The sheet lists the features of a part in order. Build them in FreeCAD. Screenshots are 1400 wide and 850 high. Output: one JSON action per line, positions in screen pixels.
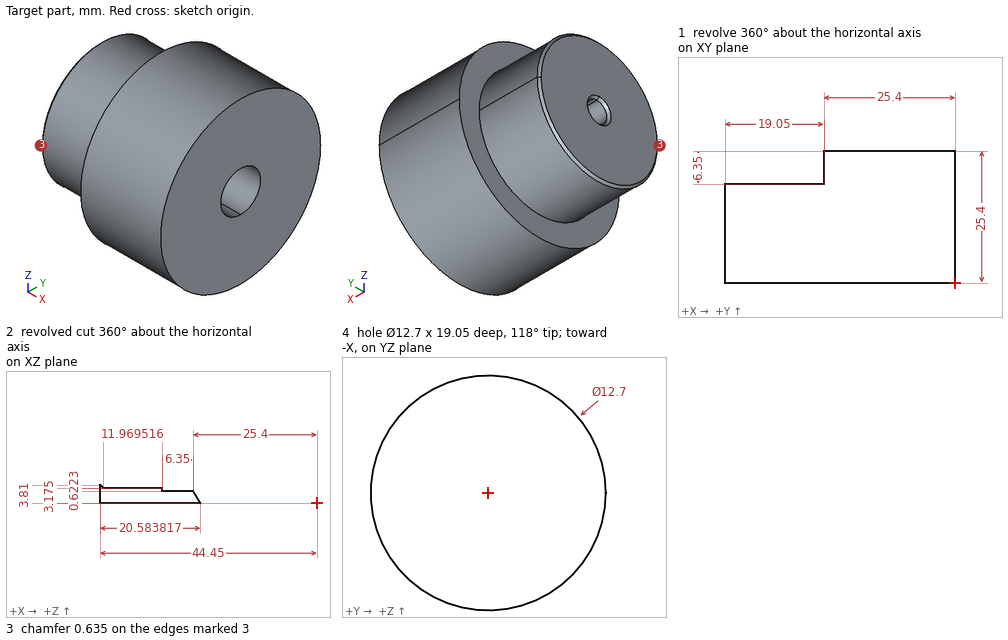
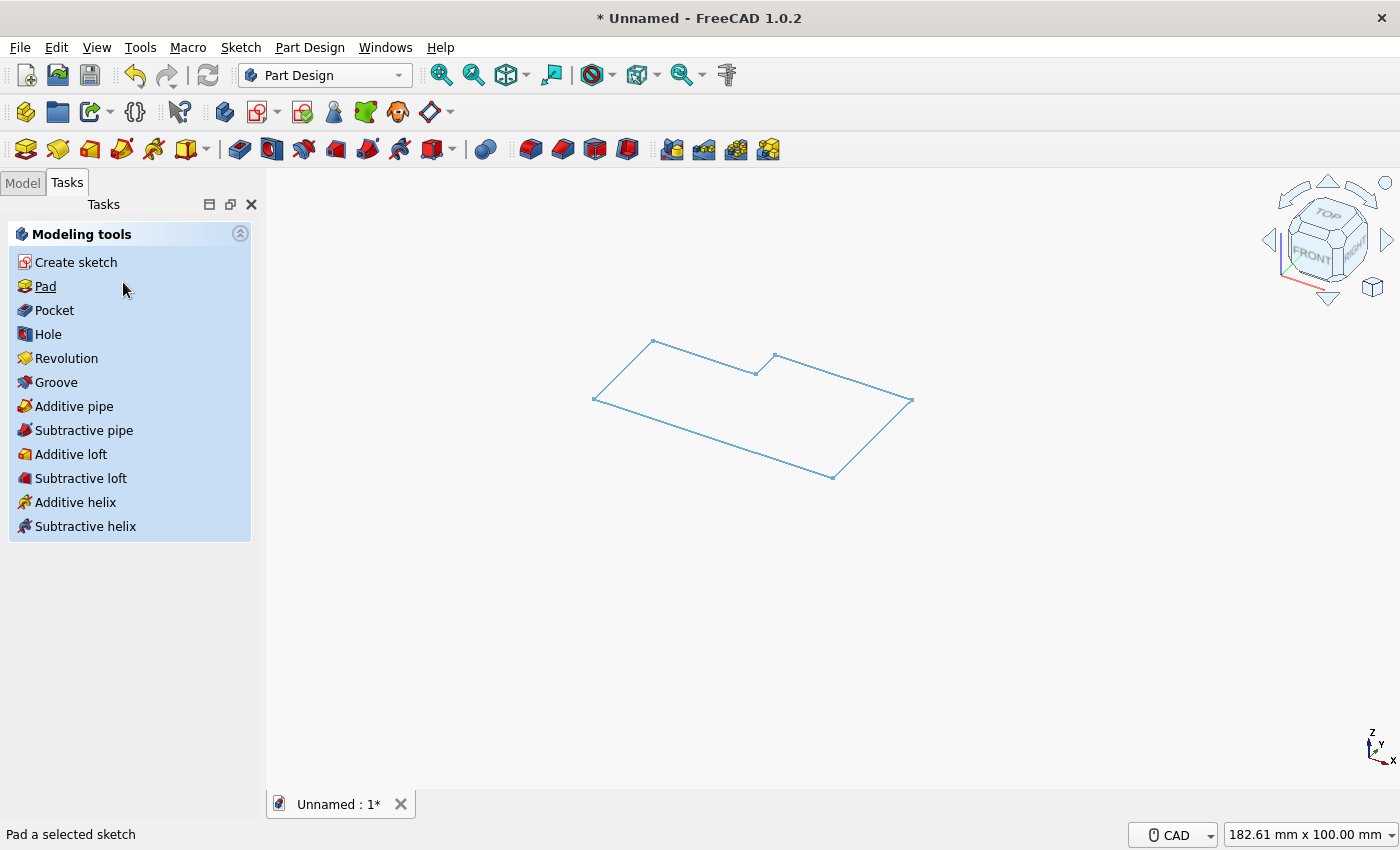
{"action": "left_click", "coordinate": [58, 150]}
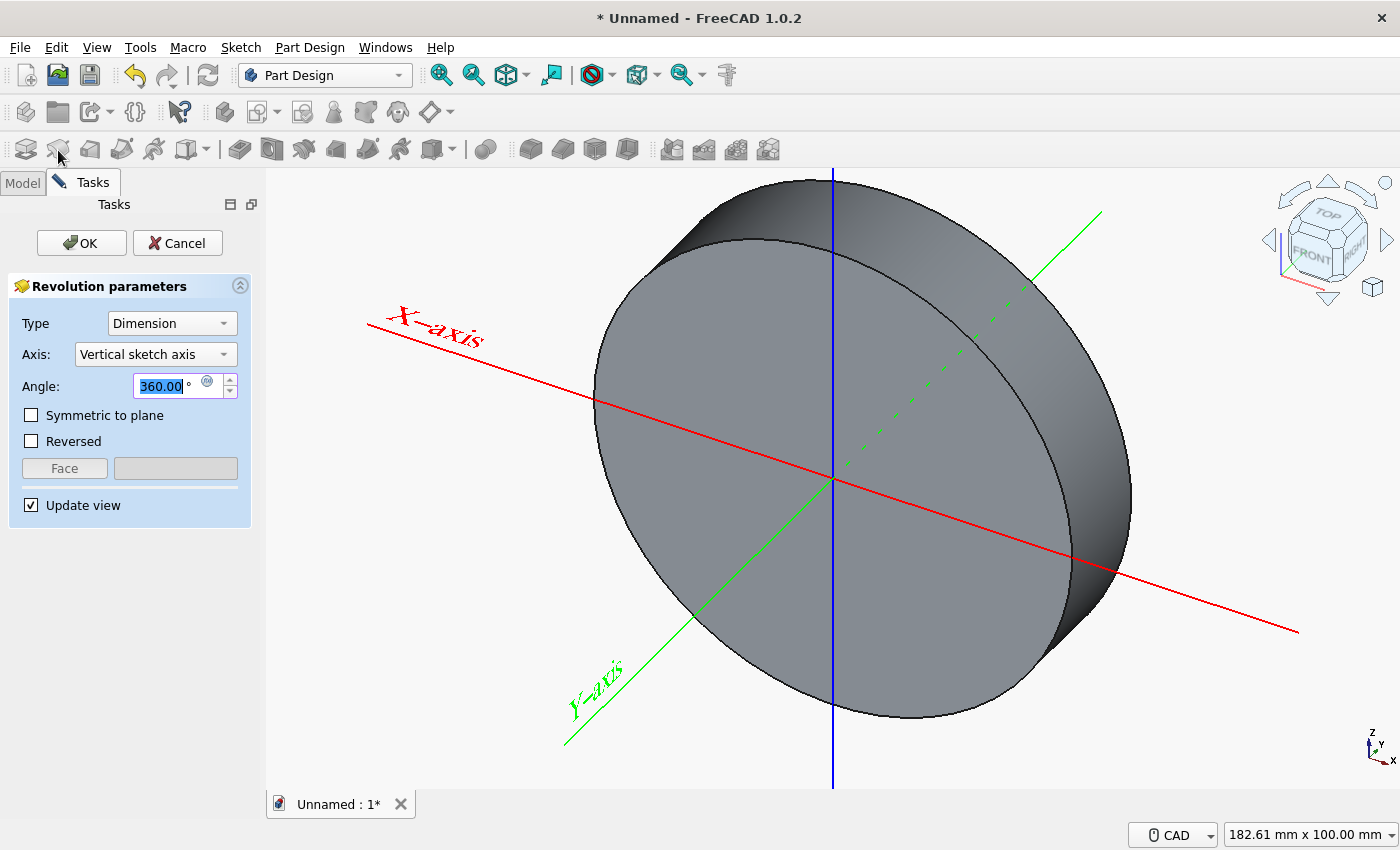
{"action": "left_click", "coordinate": [156, 354]}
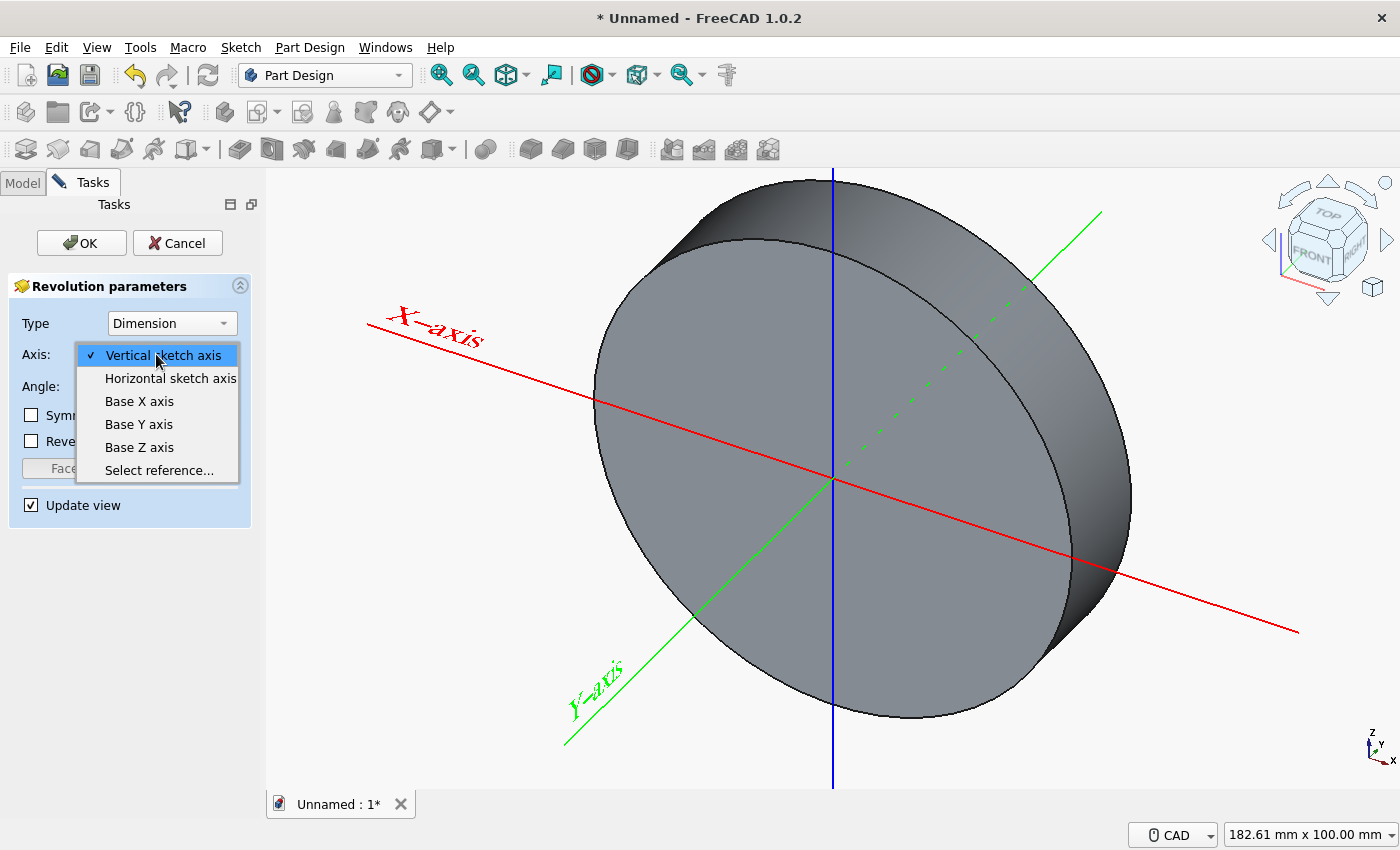
{"action": "left_click", "coordinate": [156, 378]}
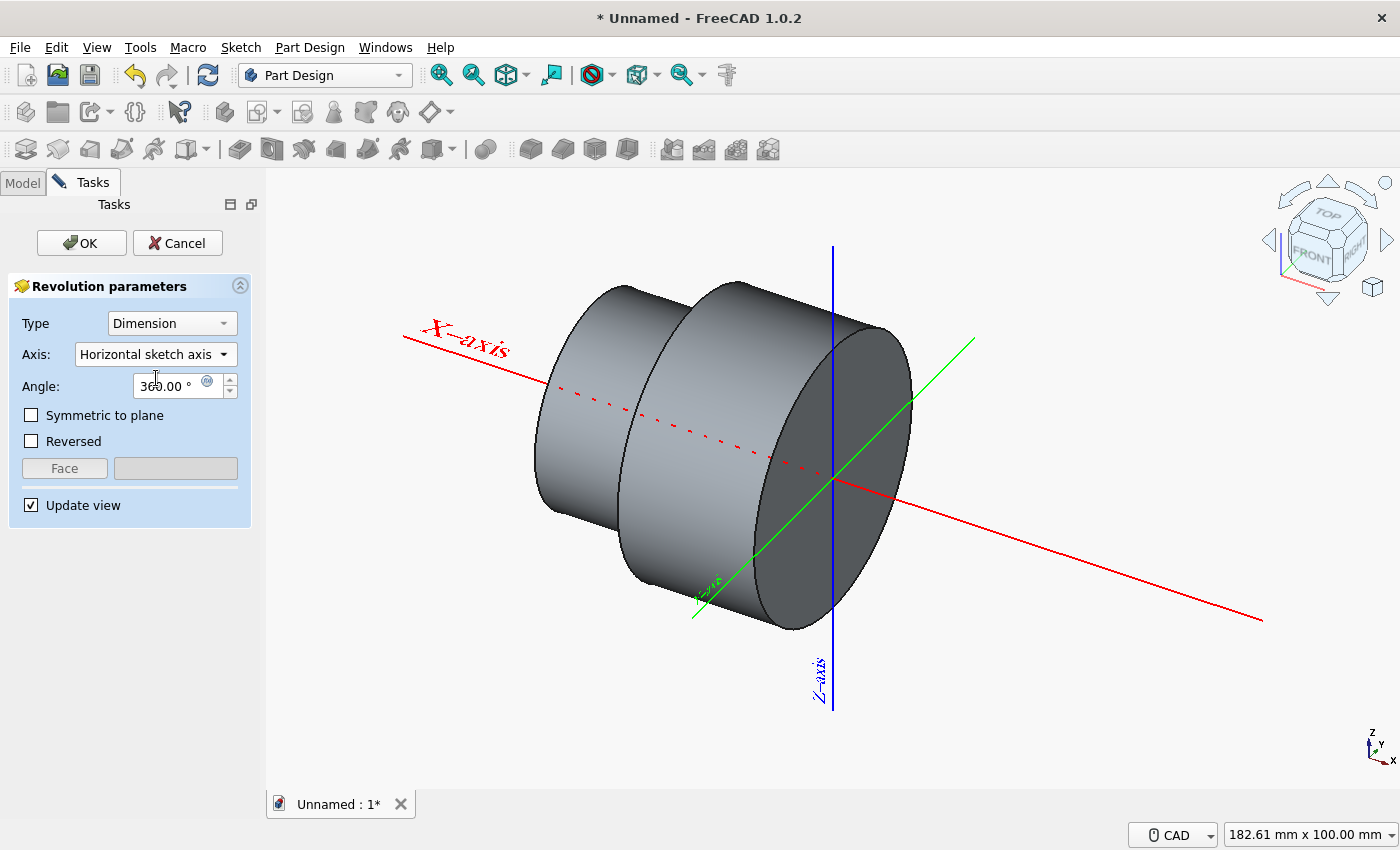
{"action": "left_click", "coordinate": [82, 243]}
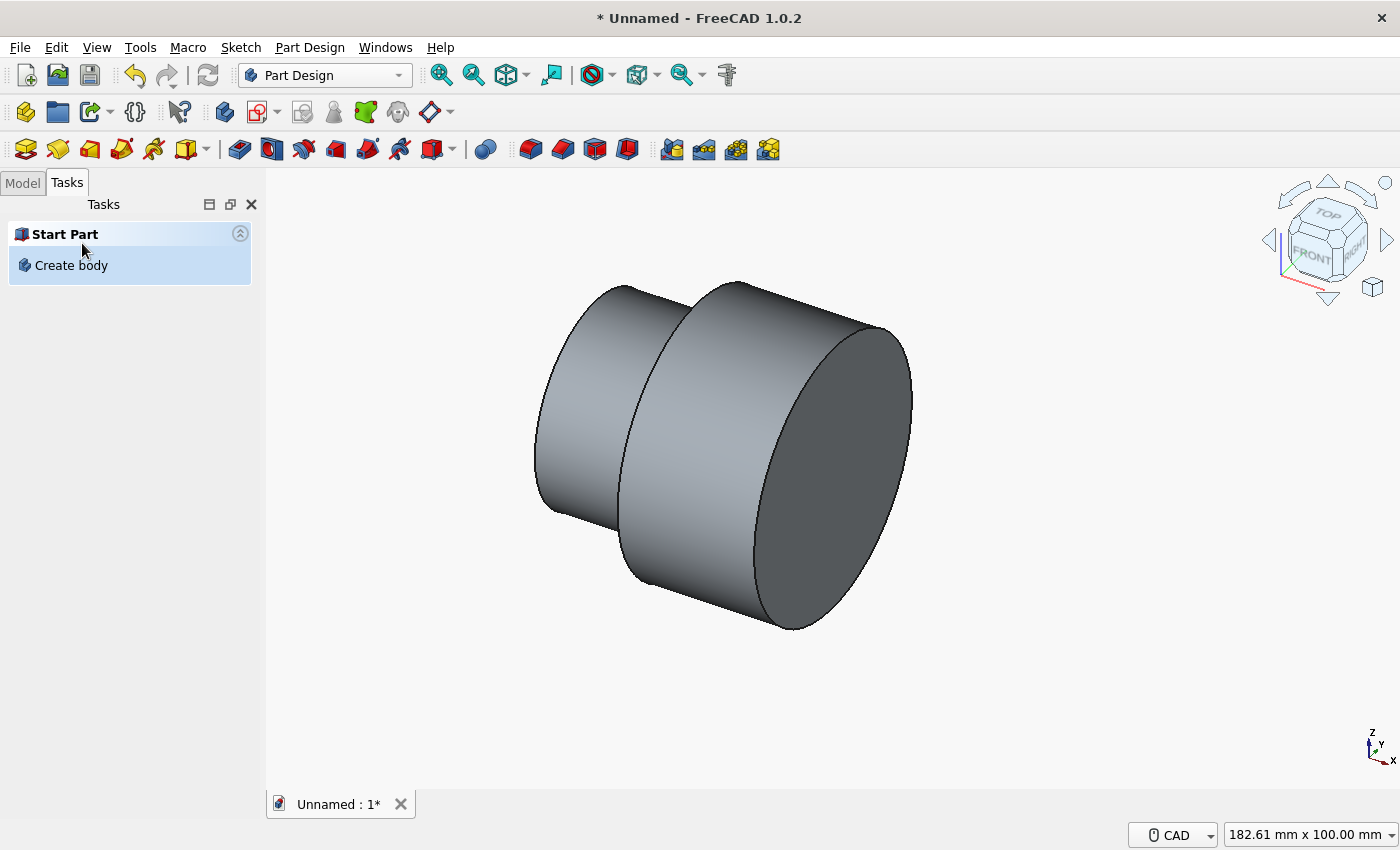
{"action": "left_click", "coordinate": [258, 112]}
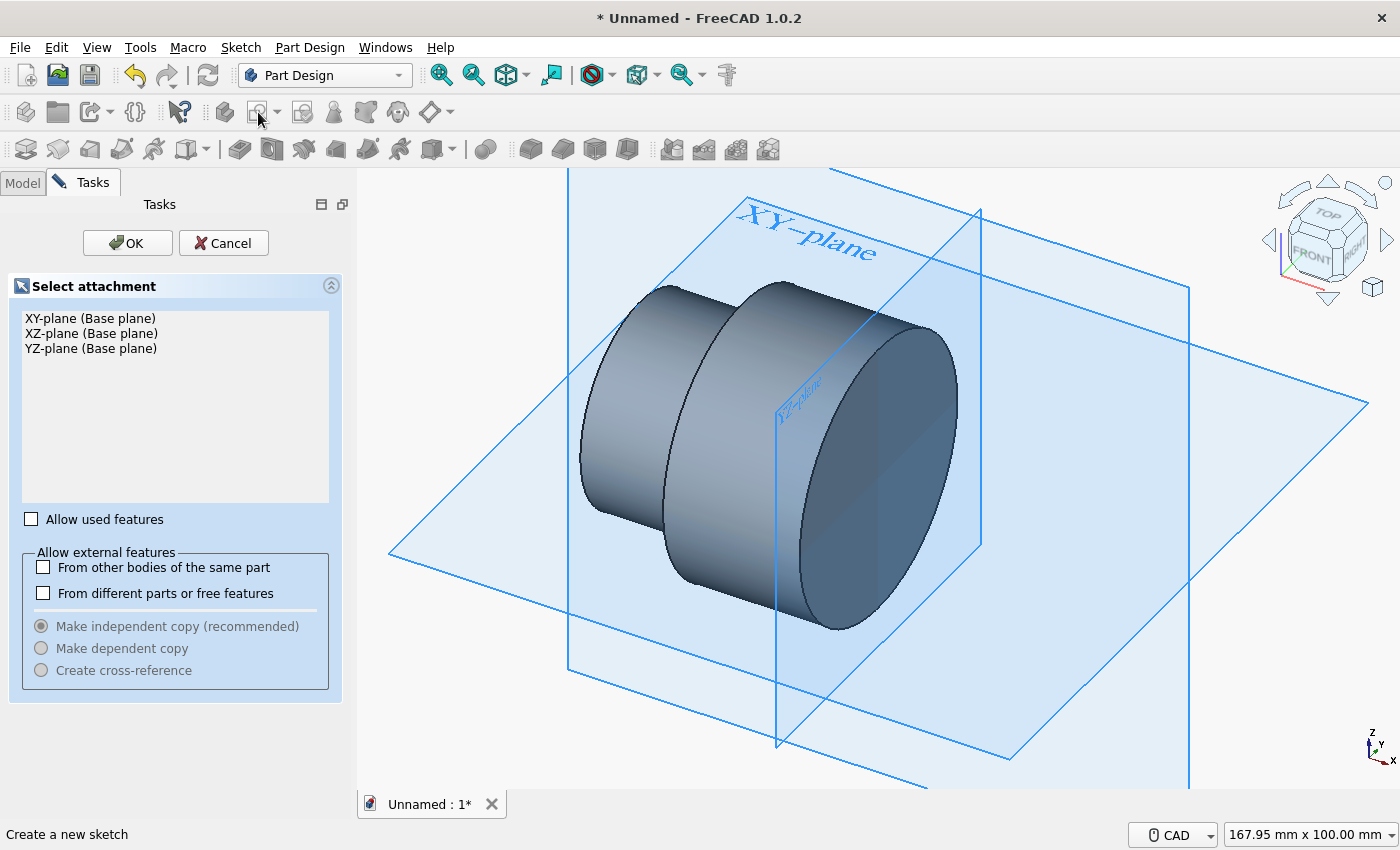
{"action": "left_click", "coordinate": [82, 334]}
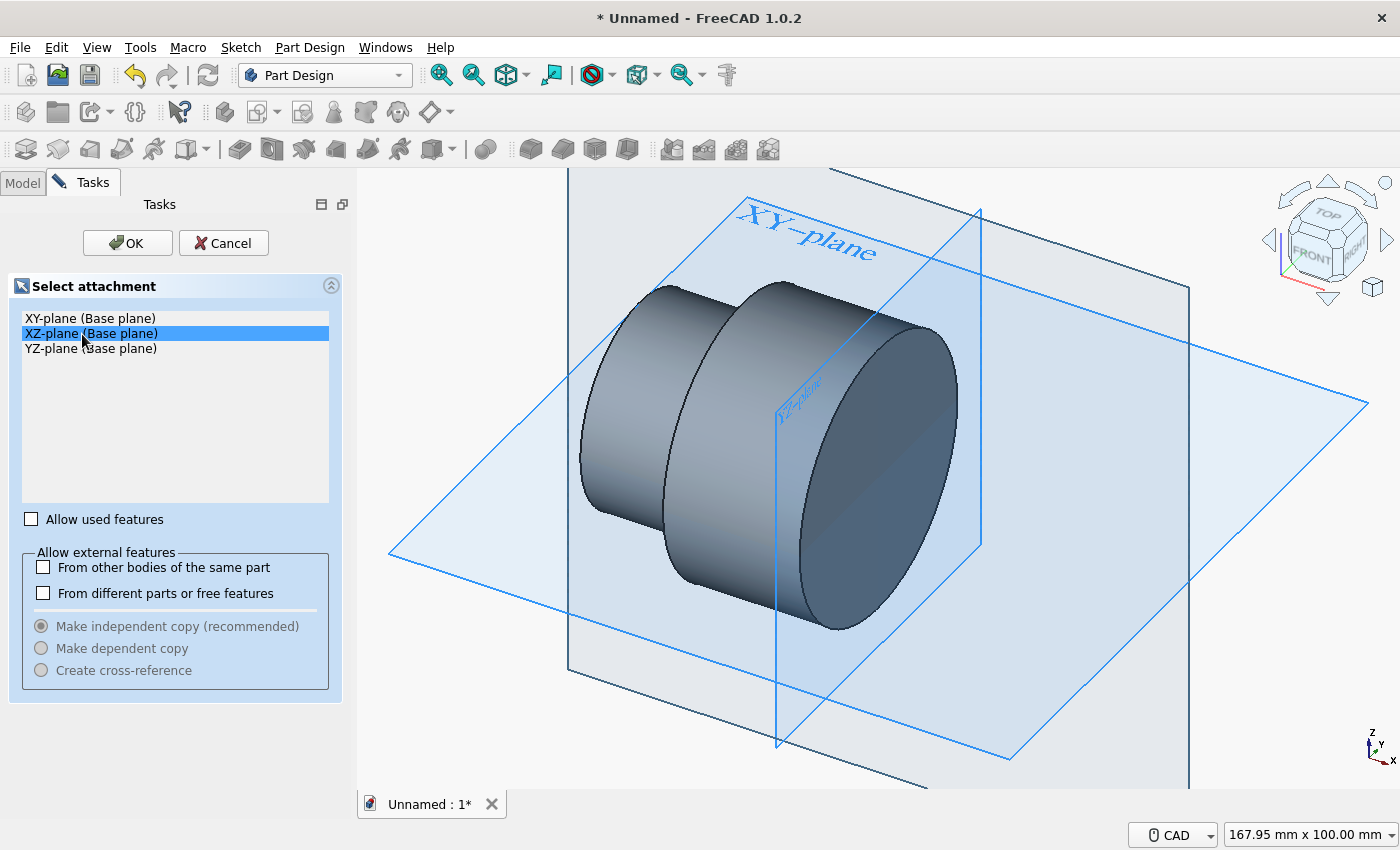
{"action": "left_click", "coordinate": [128, 243]}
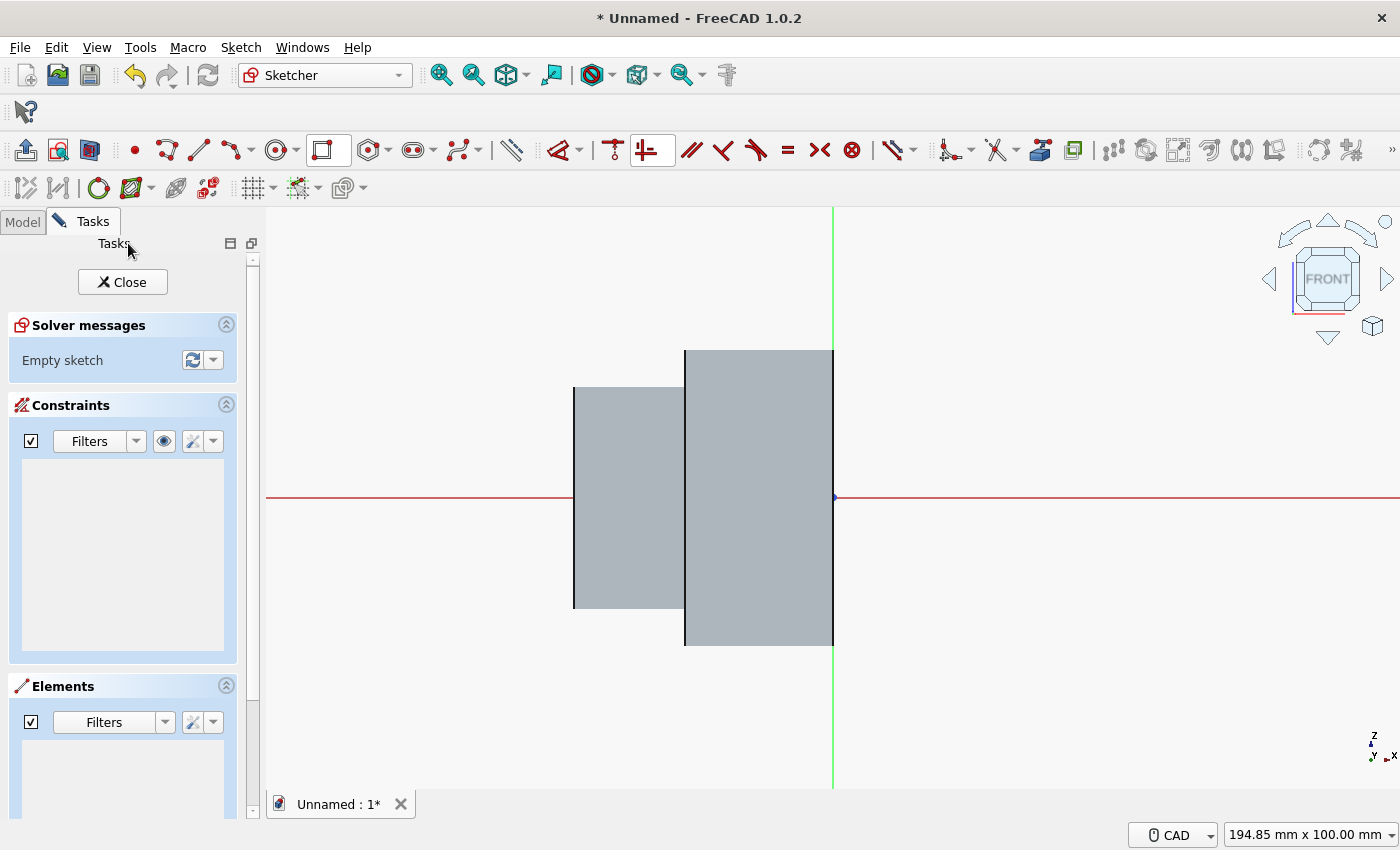
{"action": "left_click", "coordinate": [90, 150]}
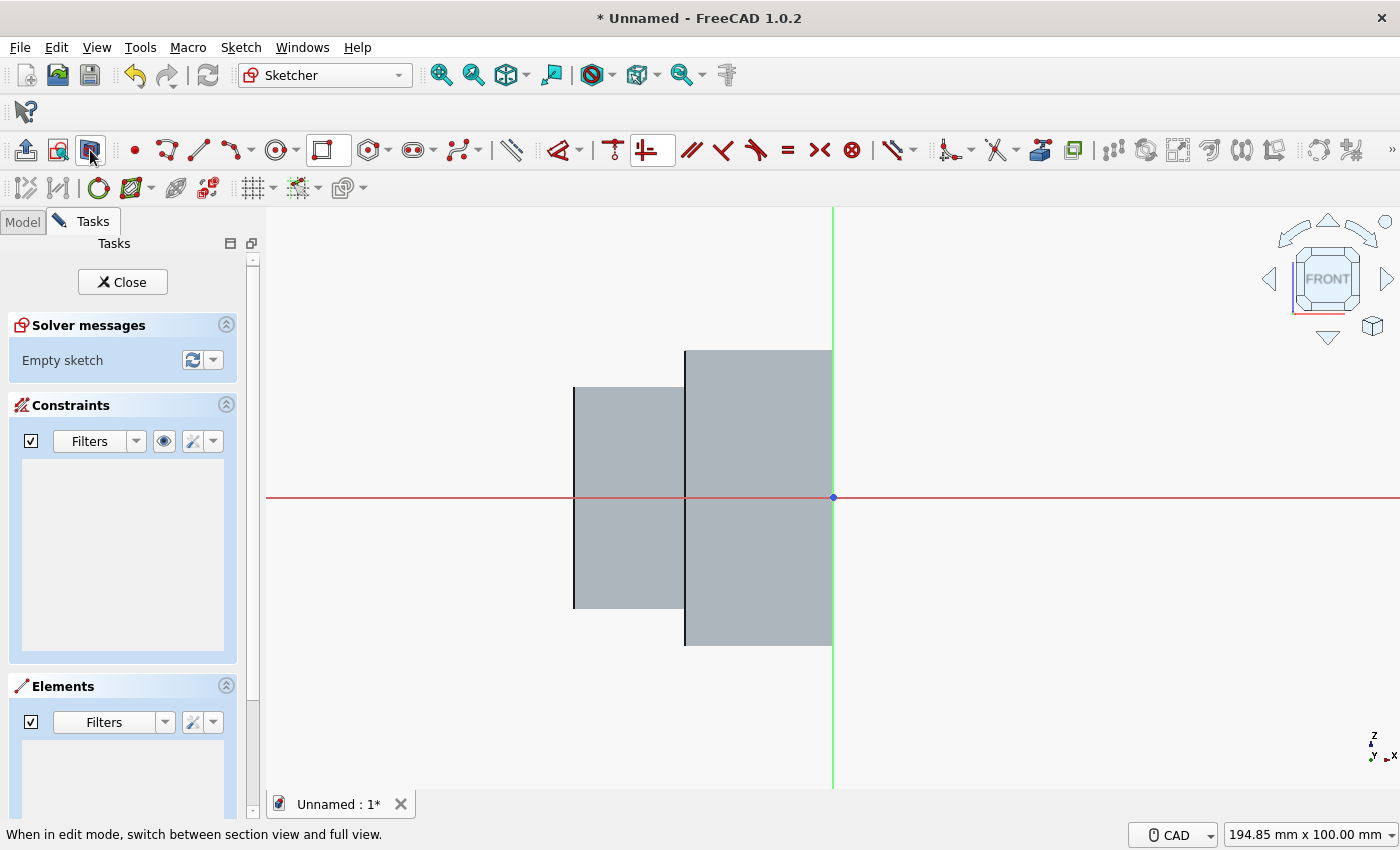
{"action": "scroll", "coordinate": [668, 480], "scroll_direction": "up", "scroll_amount": 5}